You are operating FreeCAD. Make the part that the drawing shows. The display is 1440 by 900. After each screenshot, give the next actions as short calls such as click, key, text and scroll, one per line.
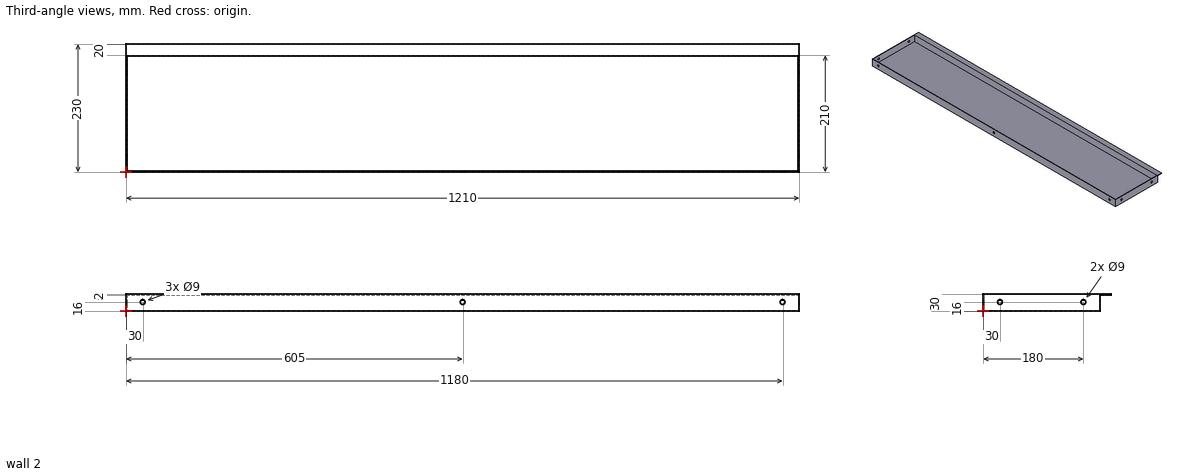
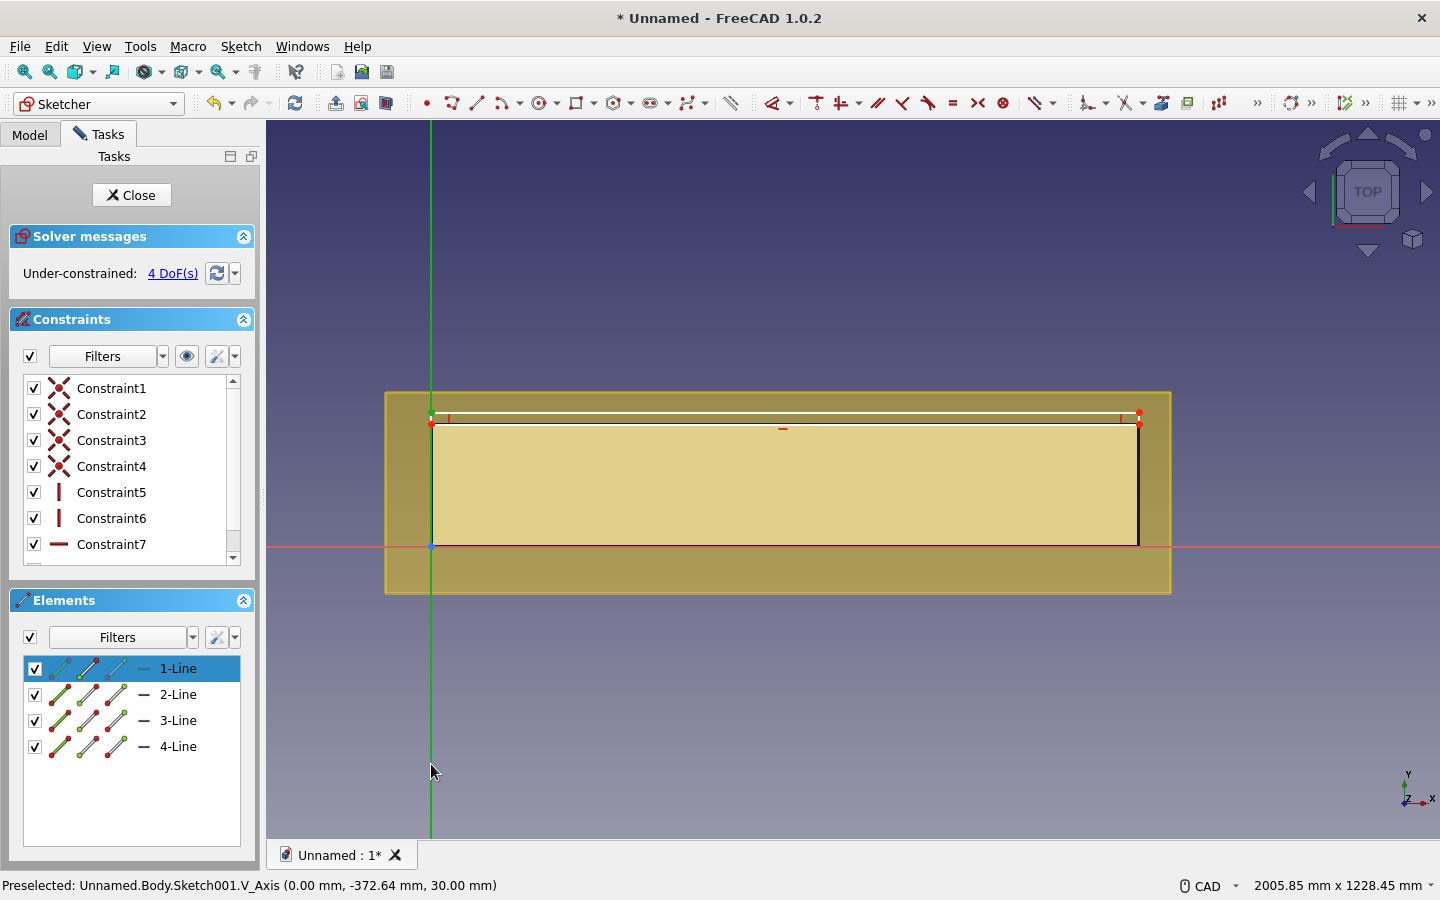
click(816, 104)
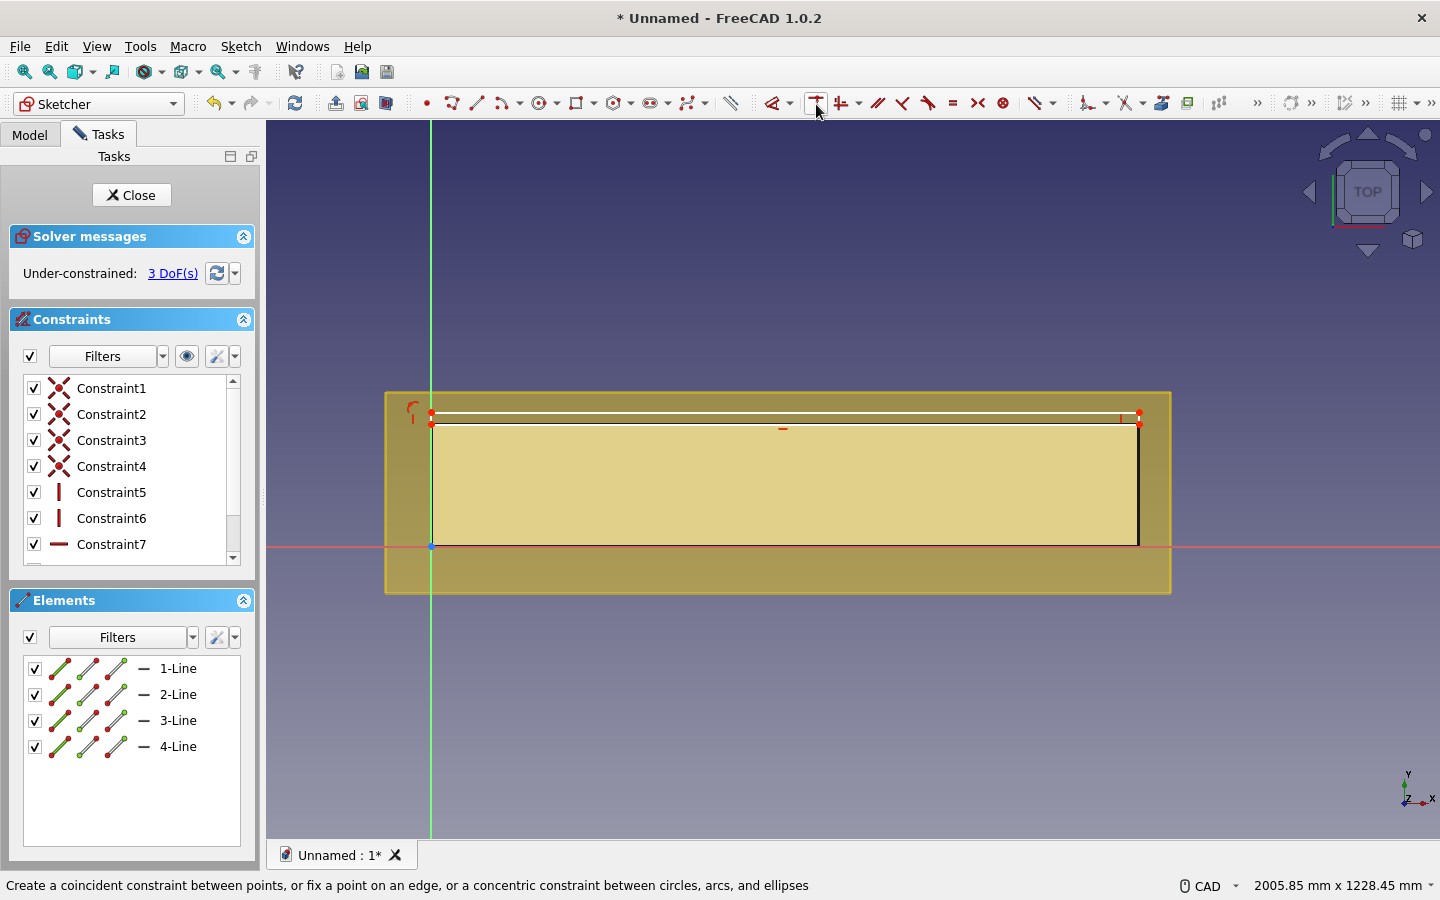
key(d)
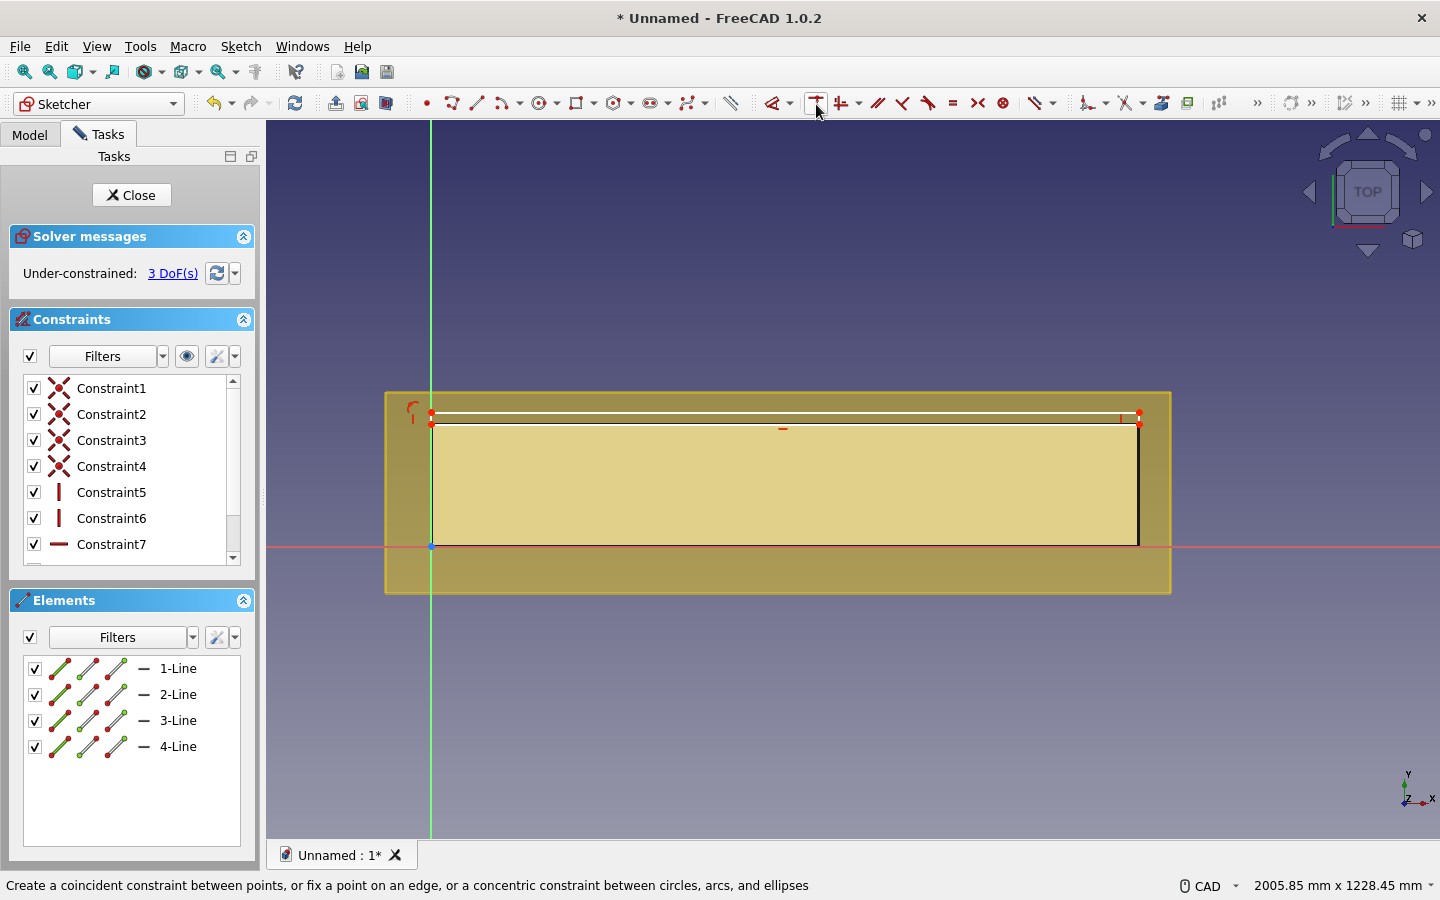
scroll(431, 419, up, 7)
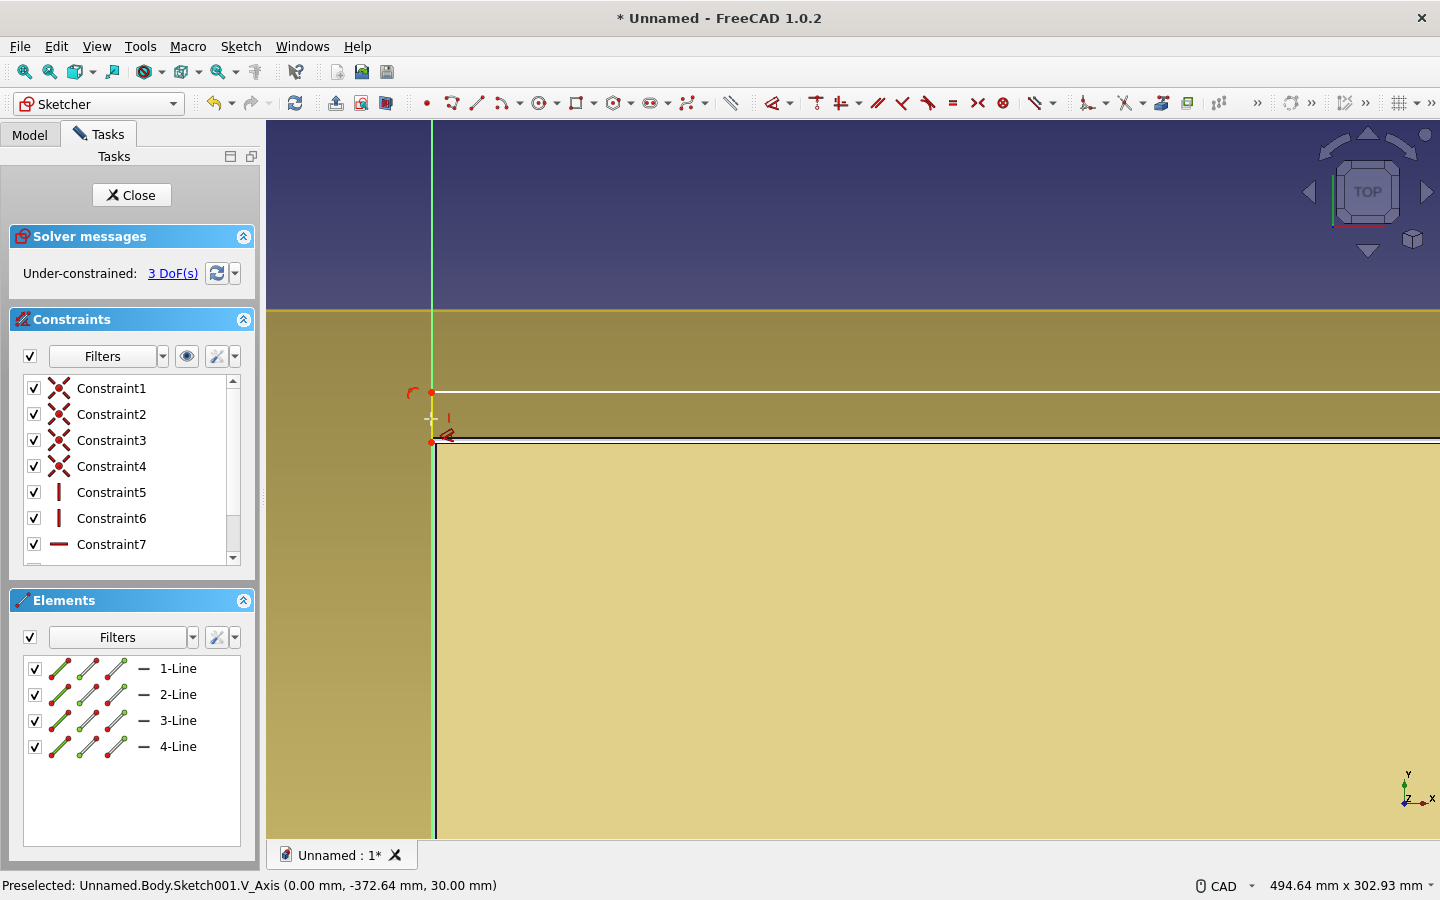
click(432, 417)
click(398, 417)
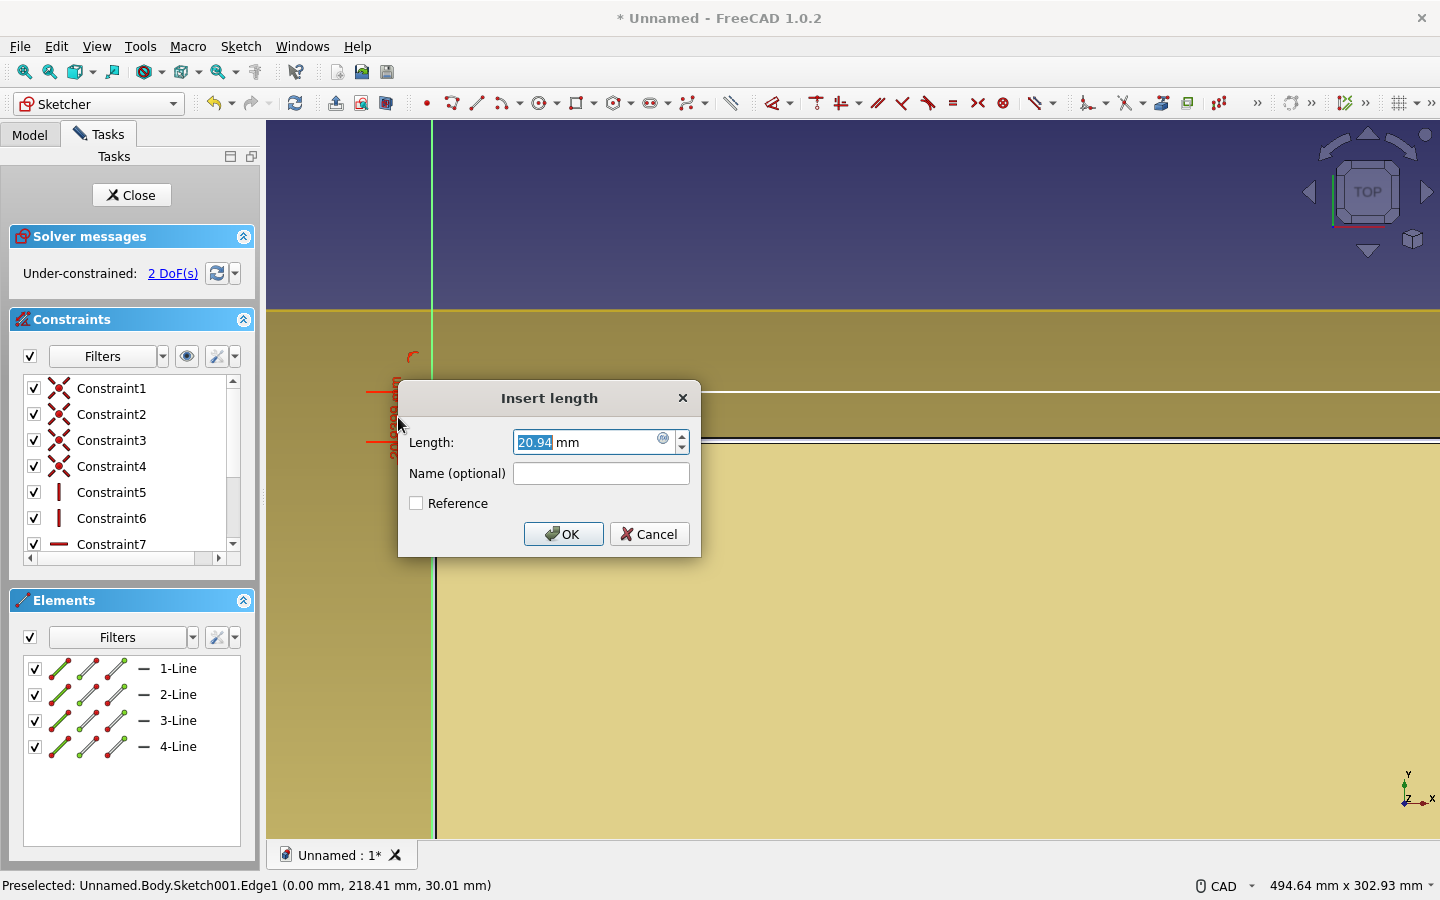
text(20)
key(Return)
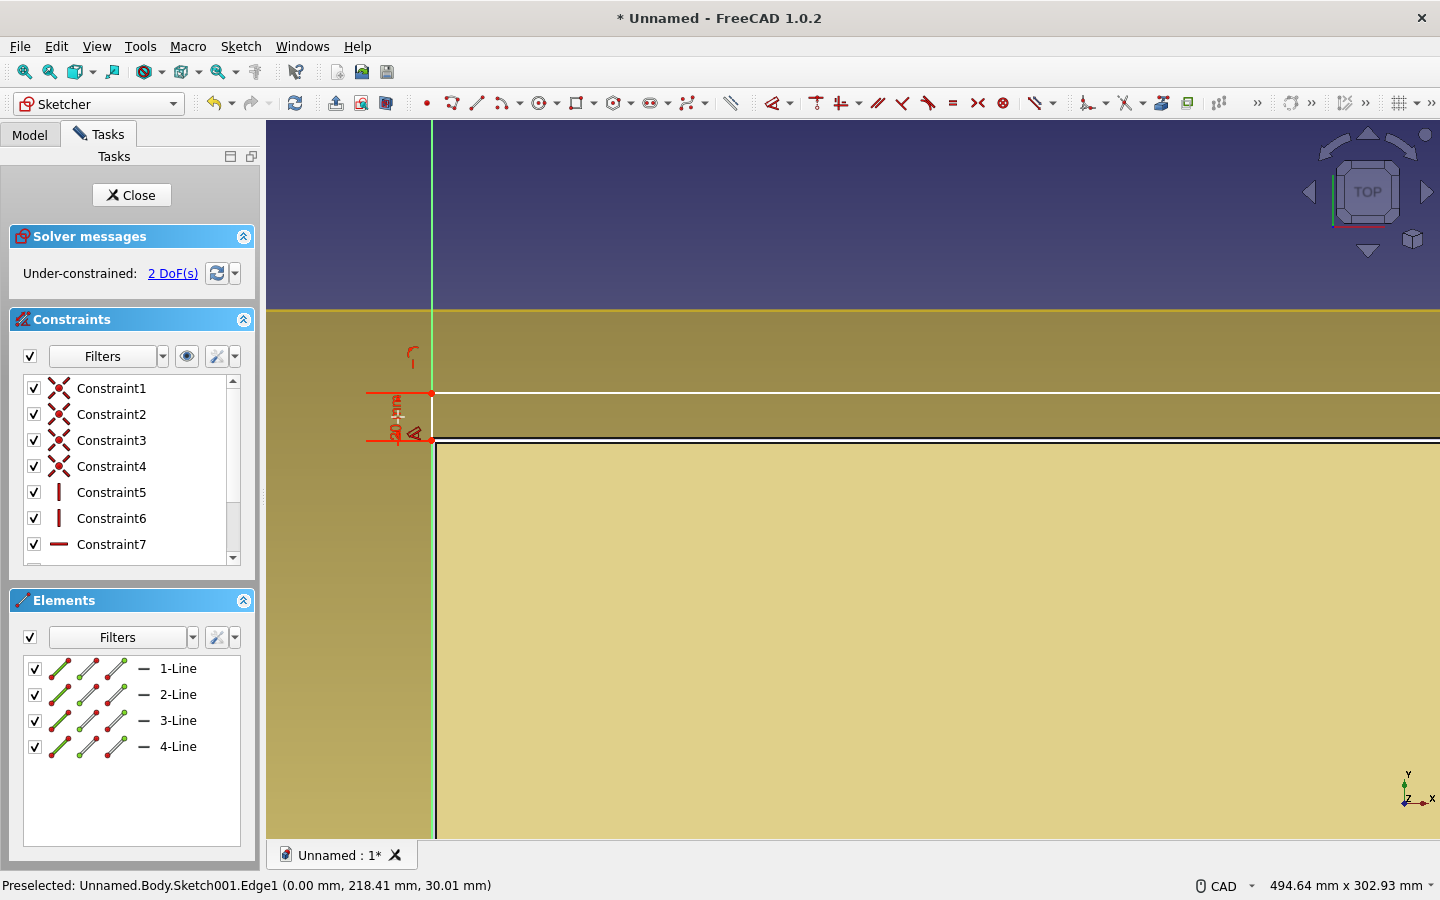
scroll(430, 419, down, 7)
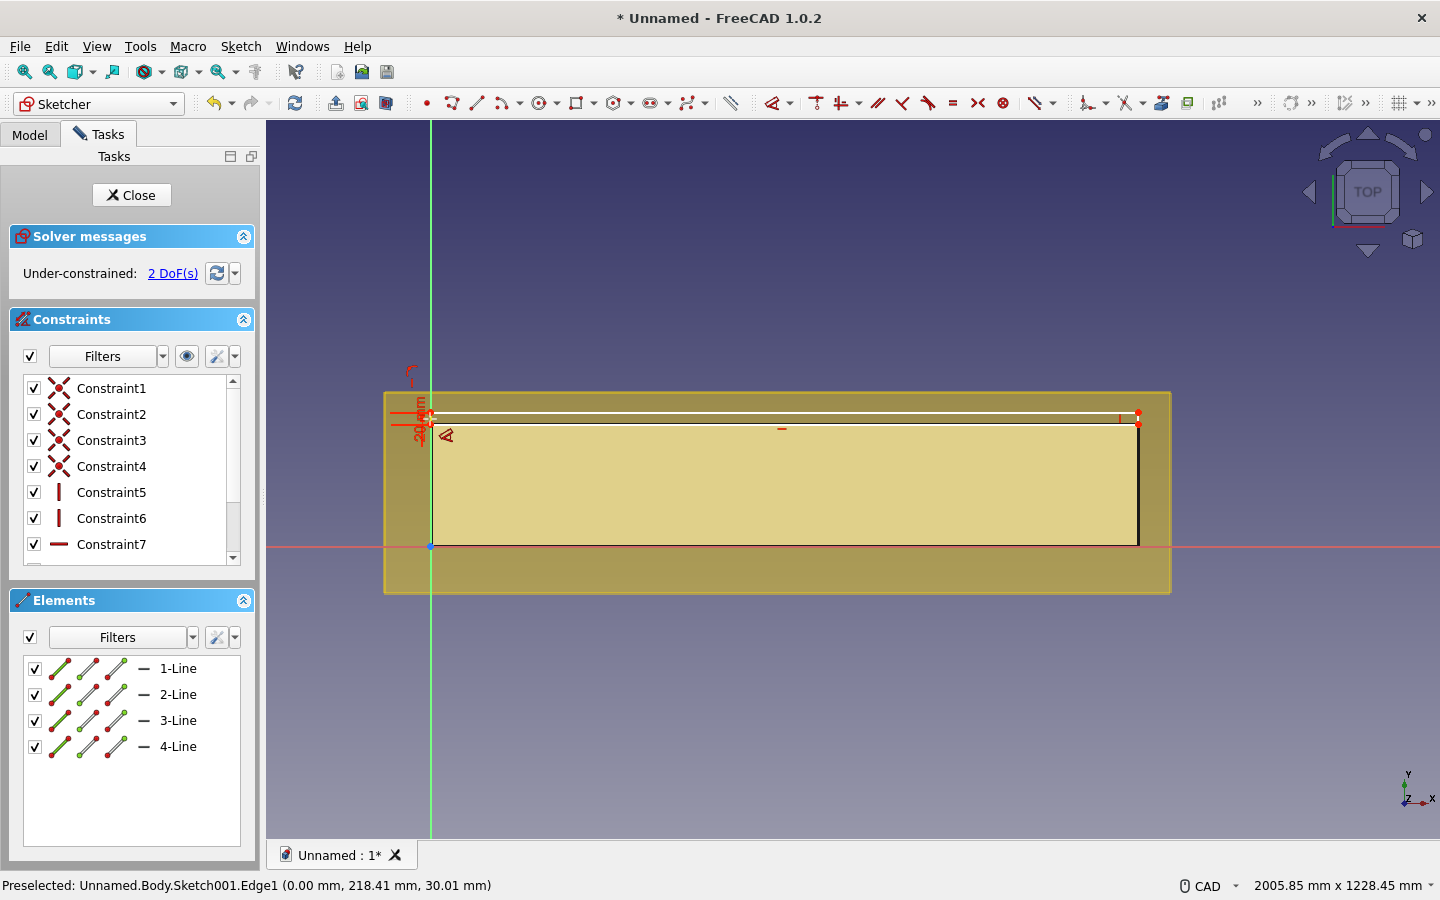
click(572, 425)
click(784, 391)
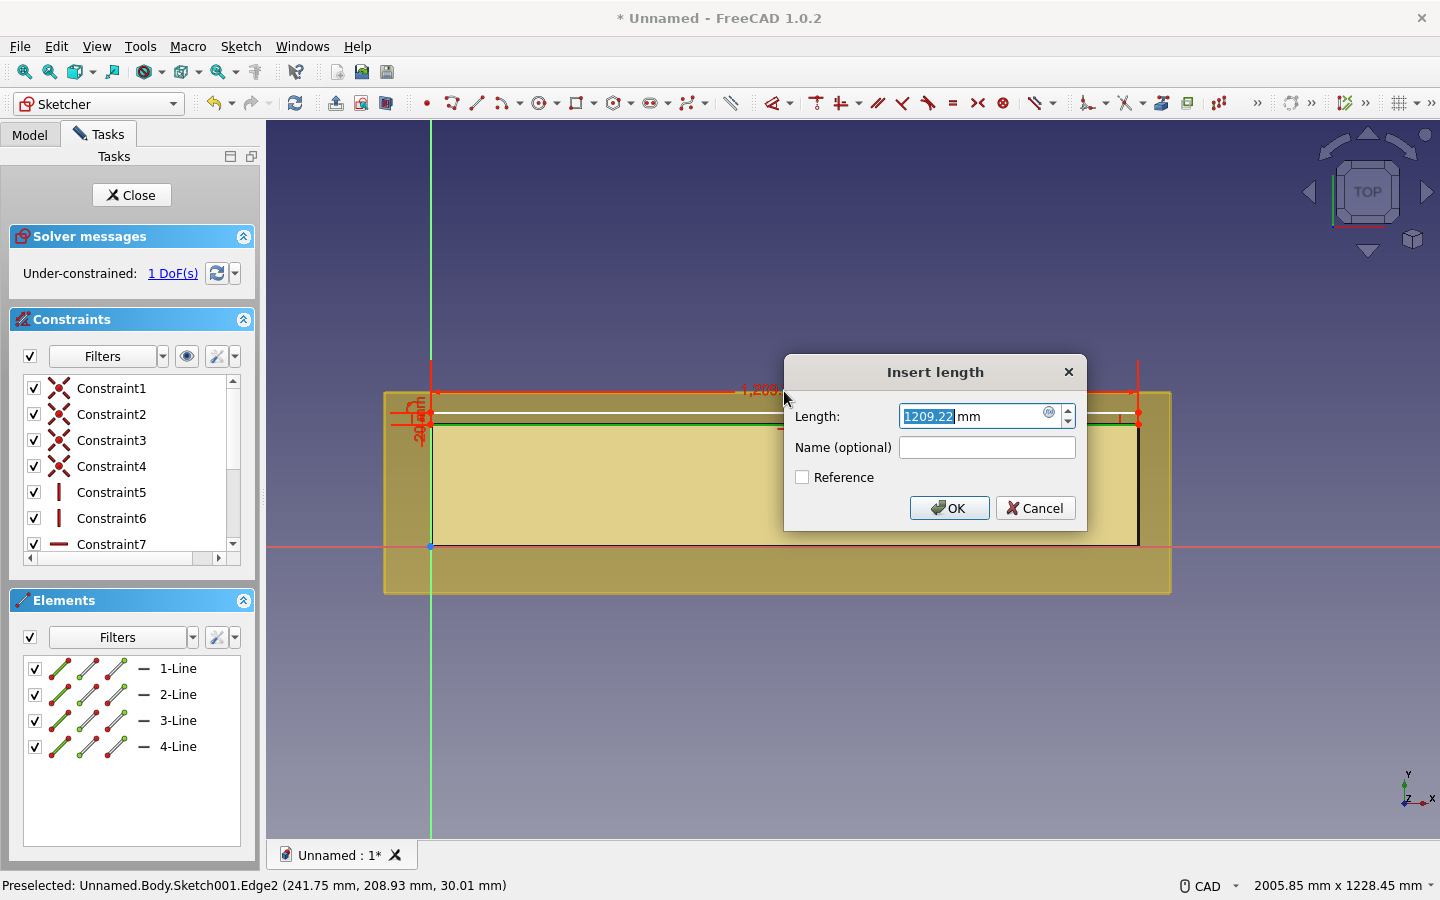
text(1210)
key(Return)